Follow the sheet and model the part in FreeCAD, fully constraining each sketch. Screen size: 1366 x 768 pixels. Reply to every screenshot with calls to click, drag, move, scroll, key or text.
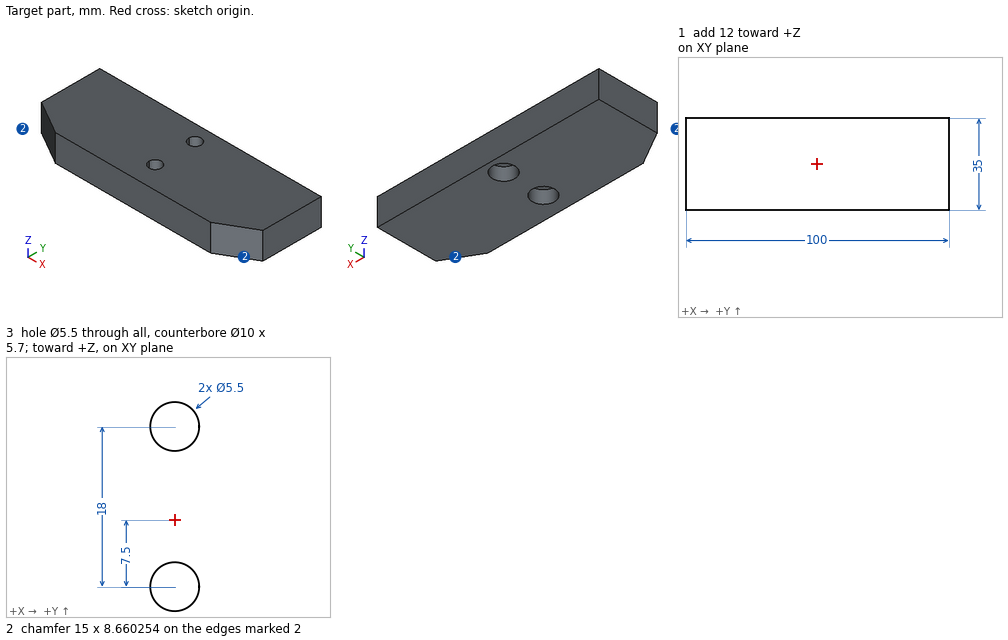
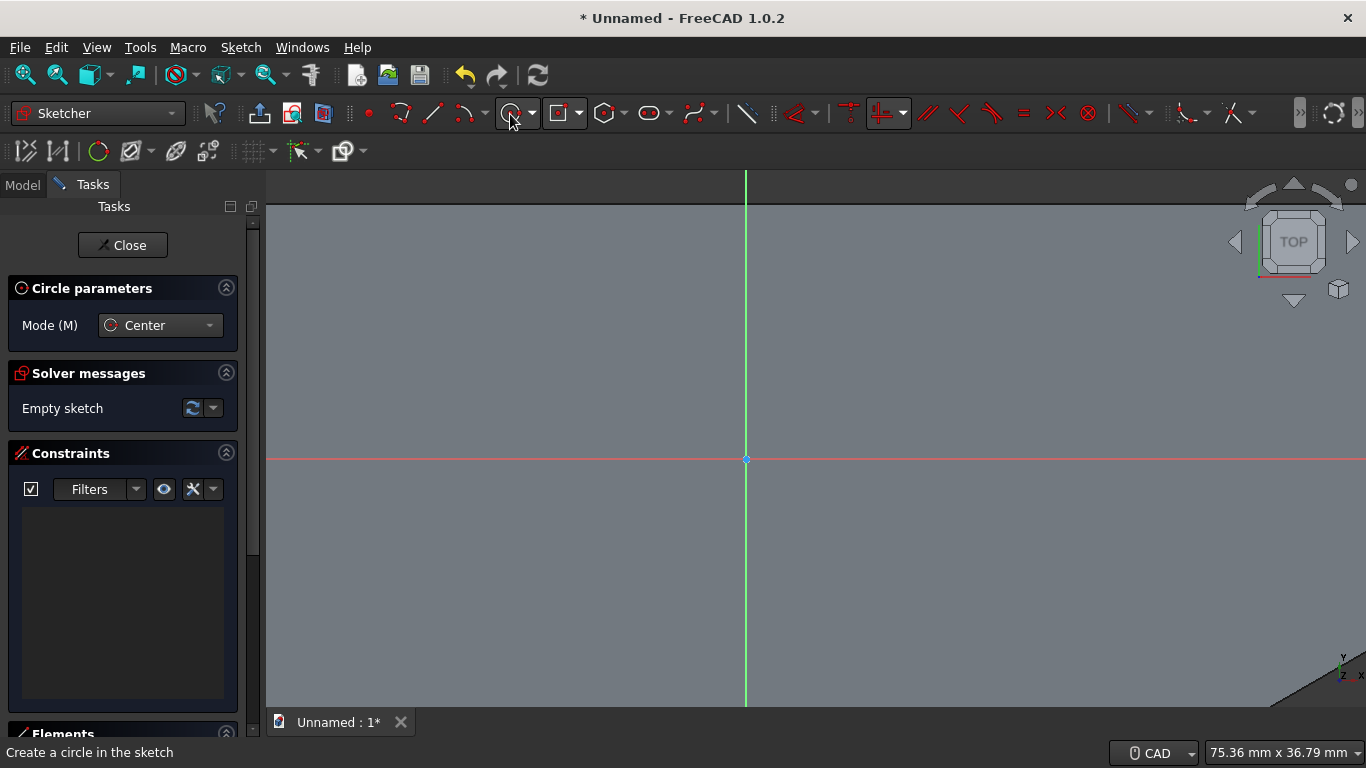
click(746, 306)
move(775, 278)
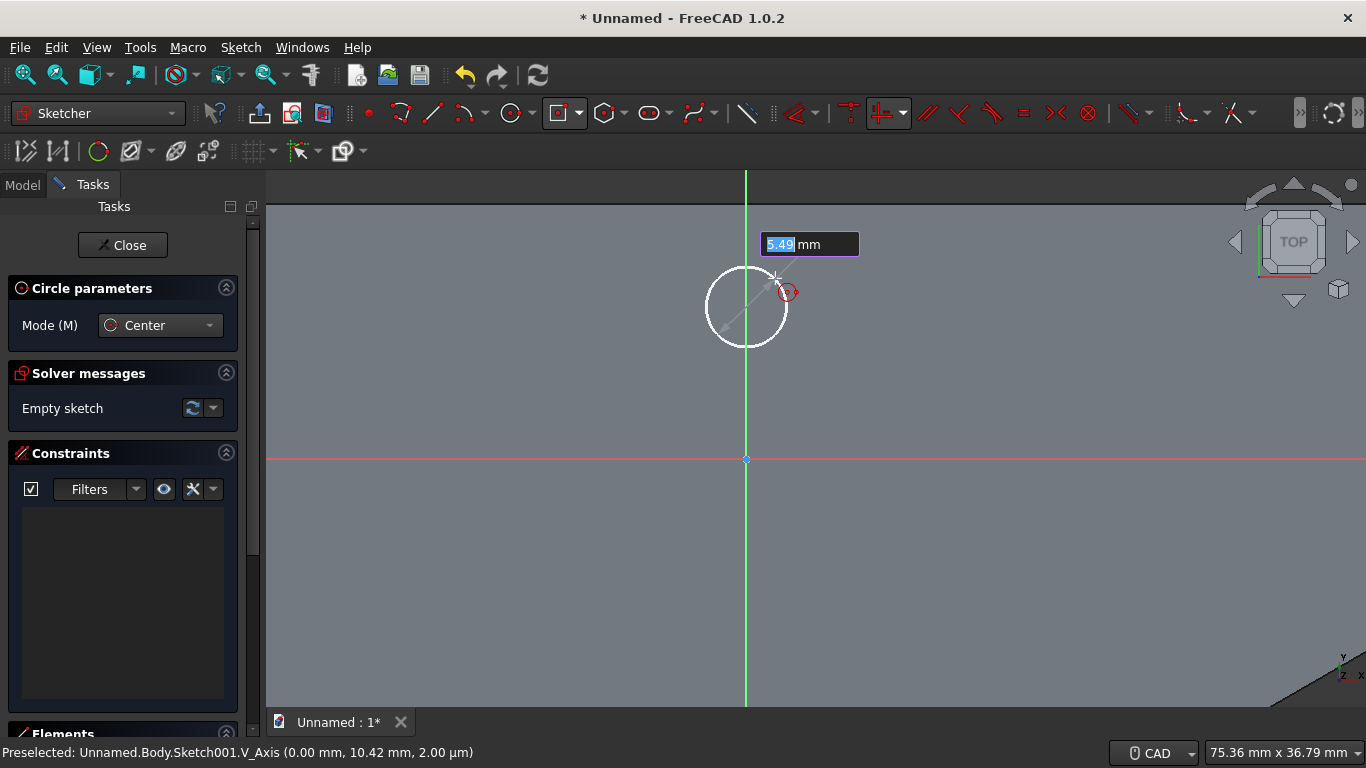
text(5.5)
key(Return)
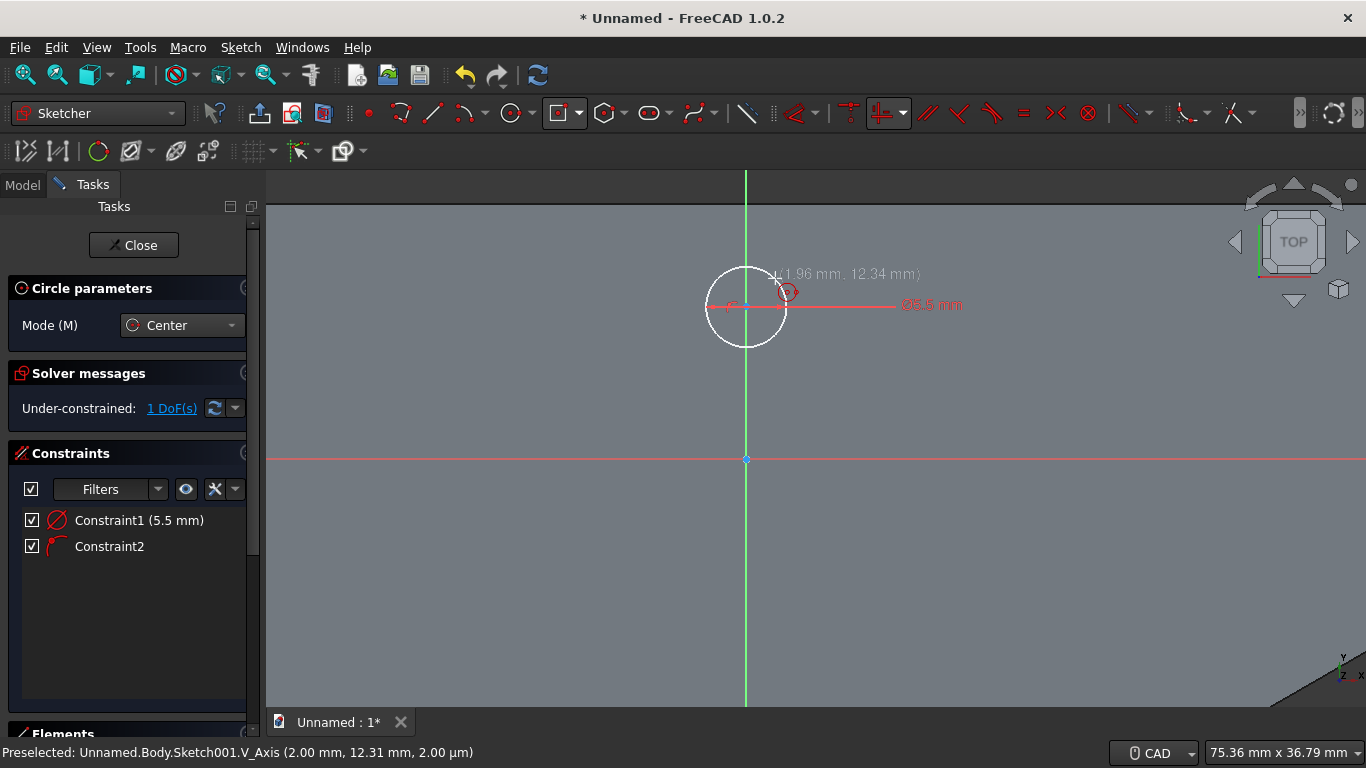
click(746, 569)
move(775, 540)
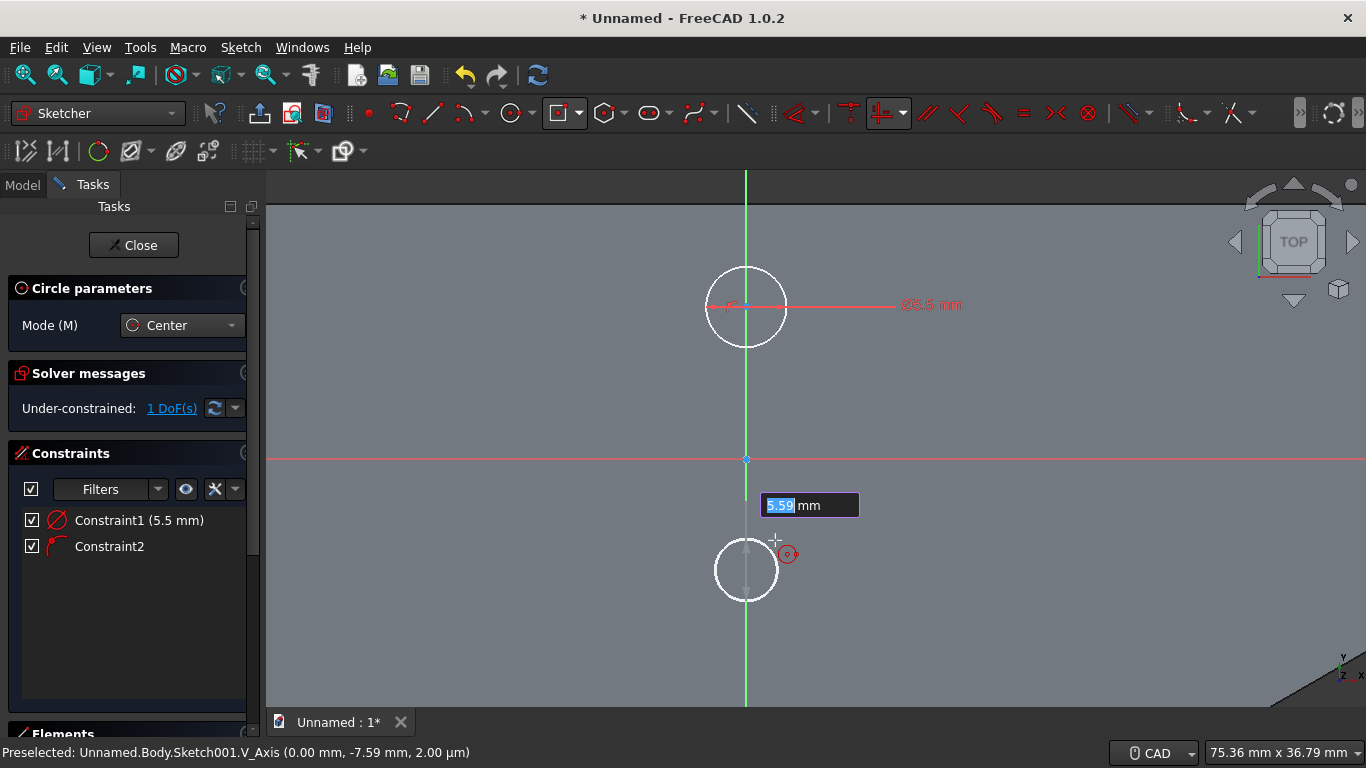
text(5.5)
key(Return)
key(Escape)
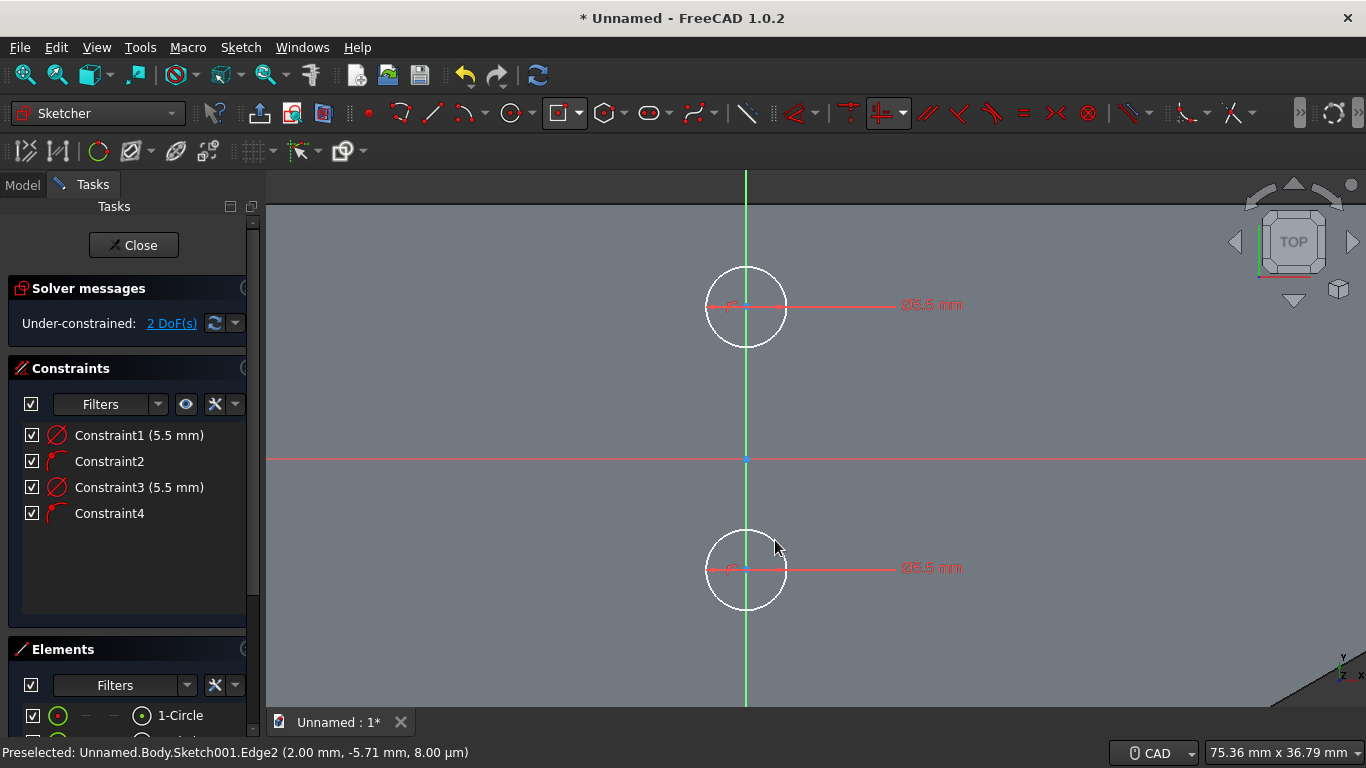
click(794, 114)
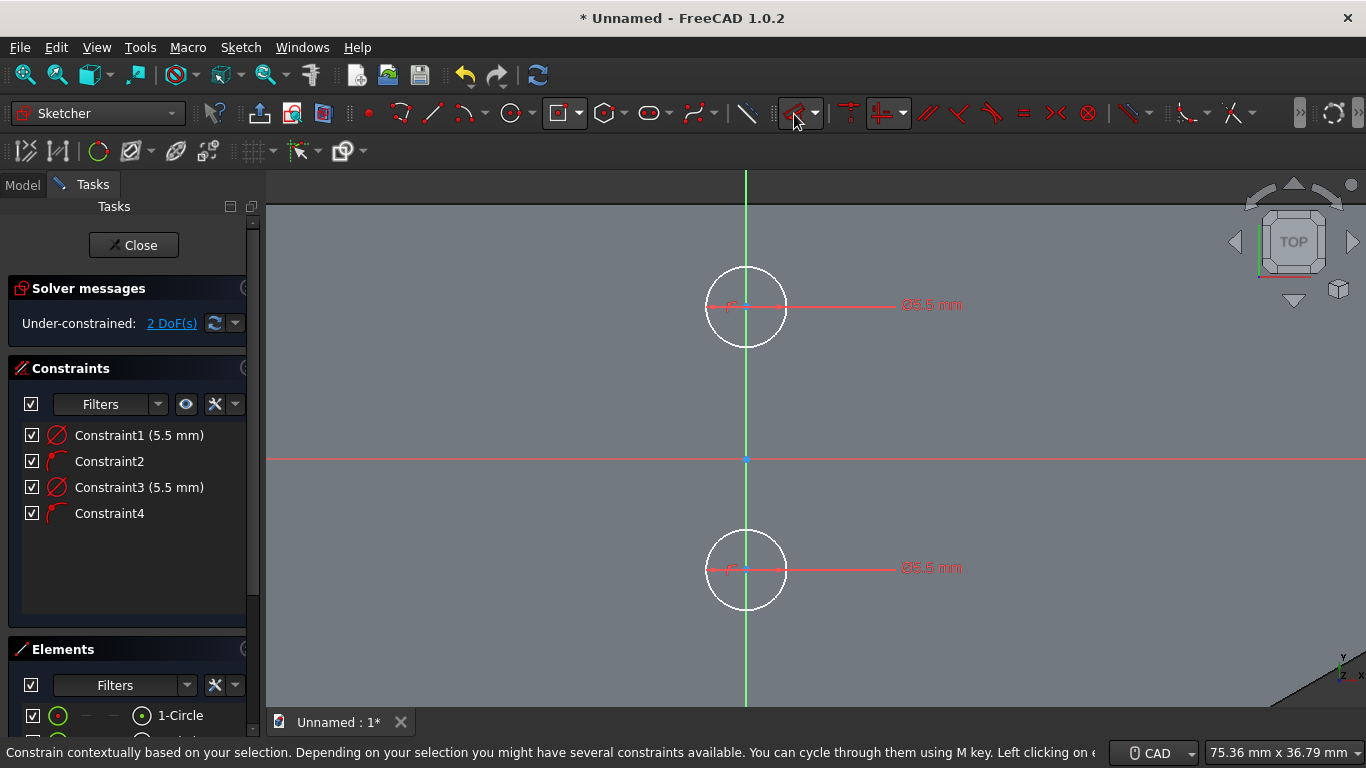
click(746, 570)
click(780, 515)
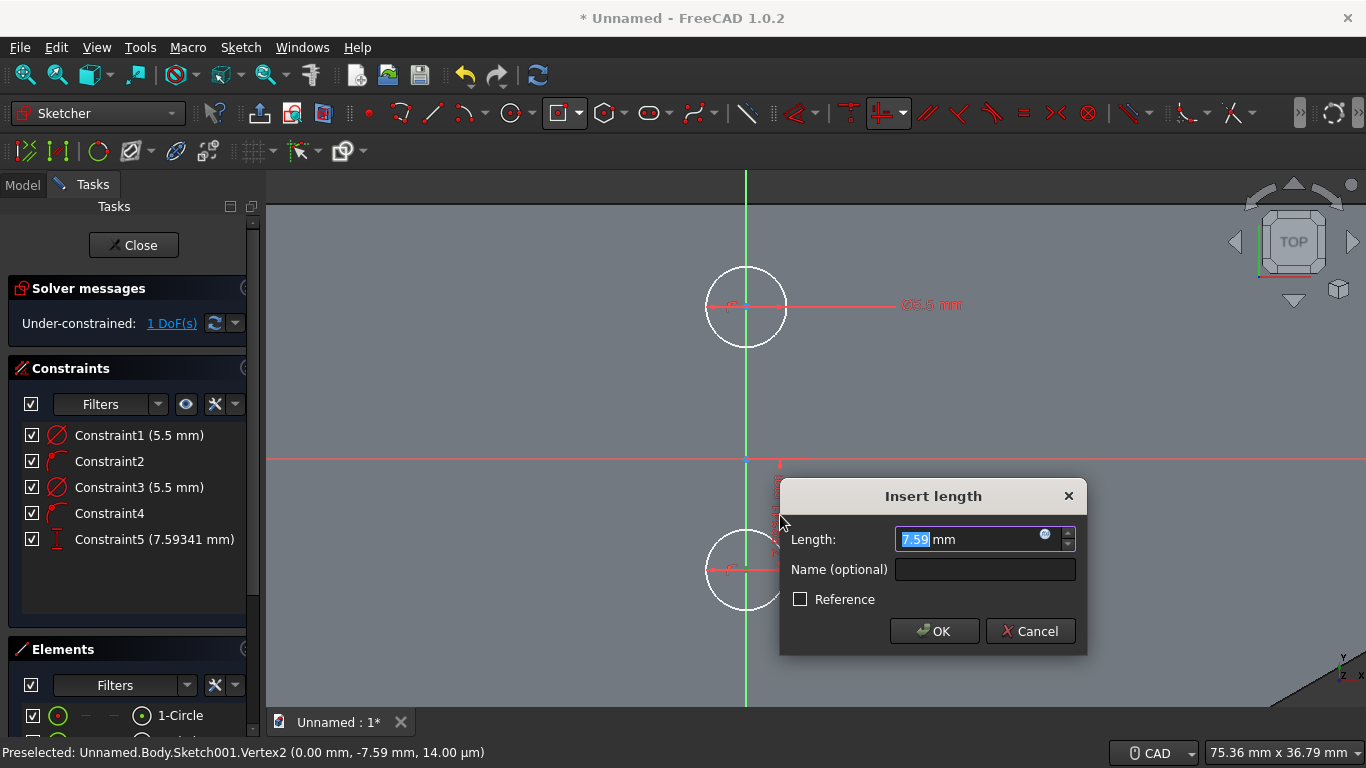
text(7.5)
key(Return)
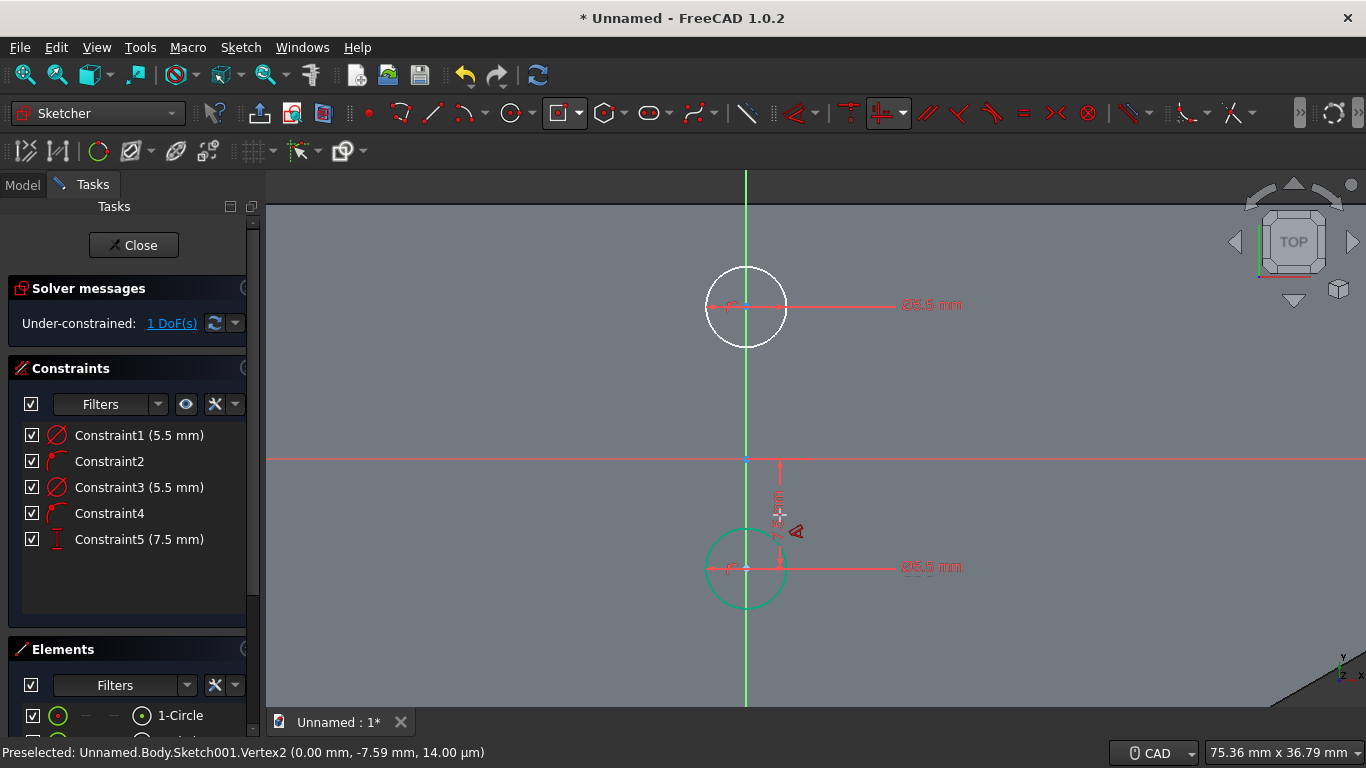
click(746, 307)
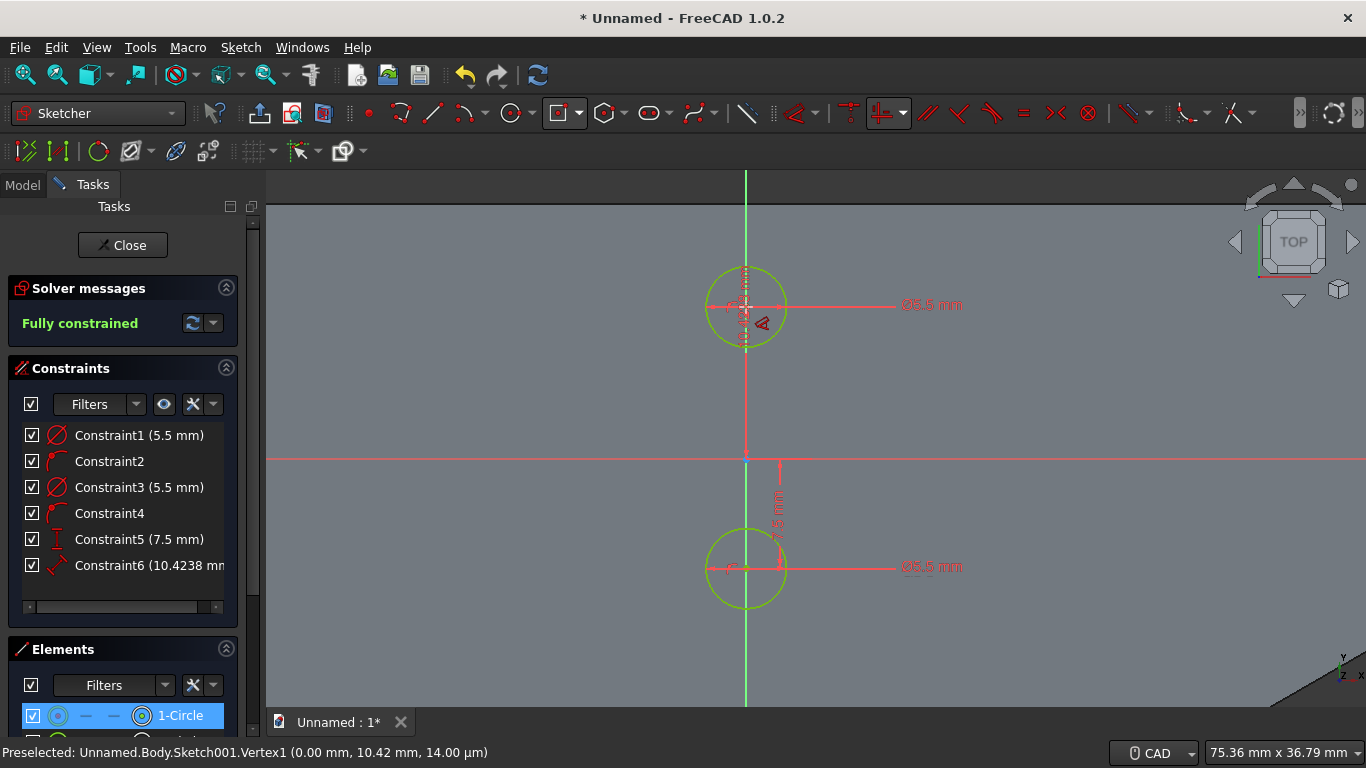
click(746, 569)
click(780, 438)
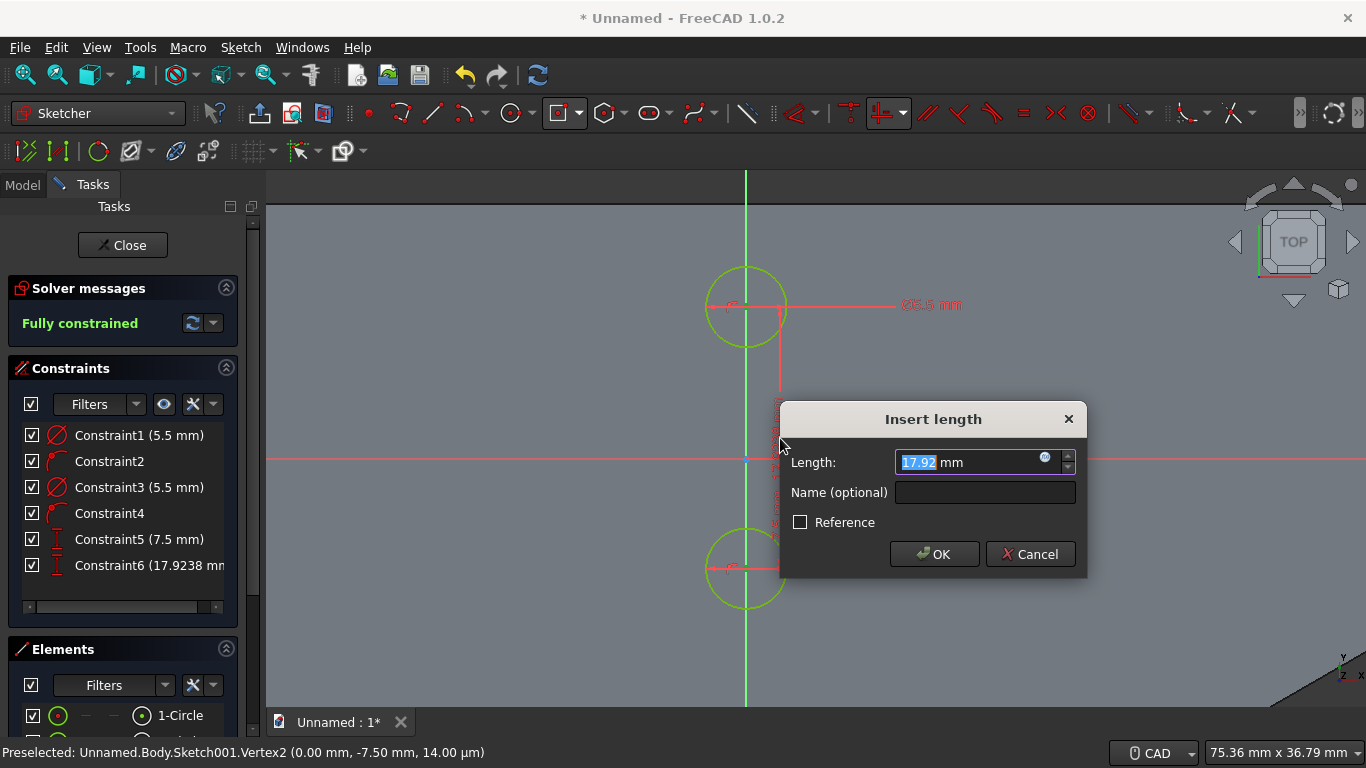
text(18)
key(Return)
key(Escape)